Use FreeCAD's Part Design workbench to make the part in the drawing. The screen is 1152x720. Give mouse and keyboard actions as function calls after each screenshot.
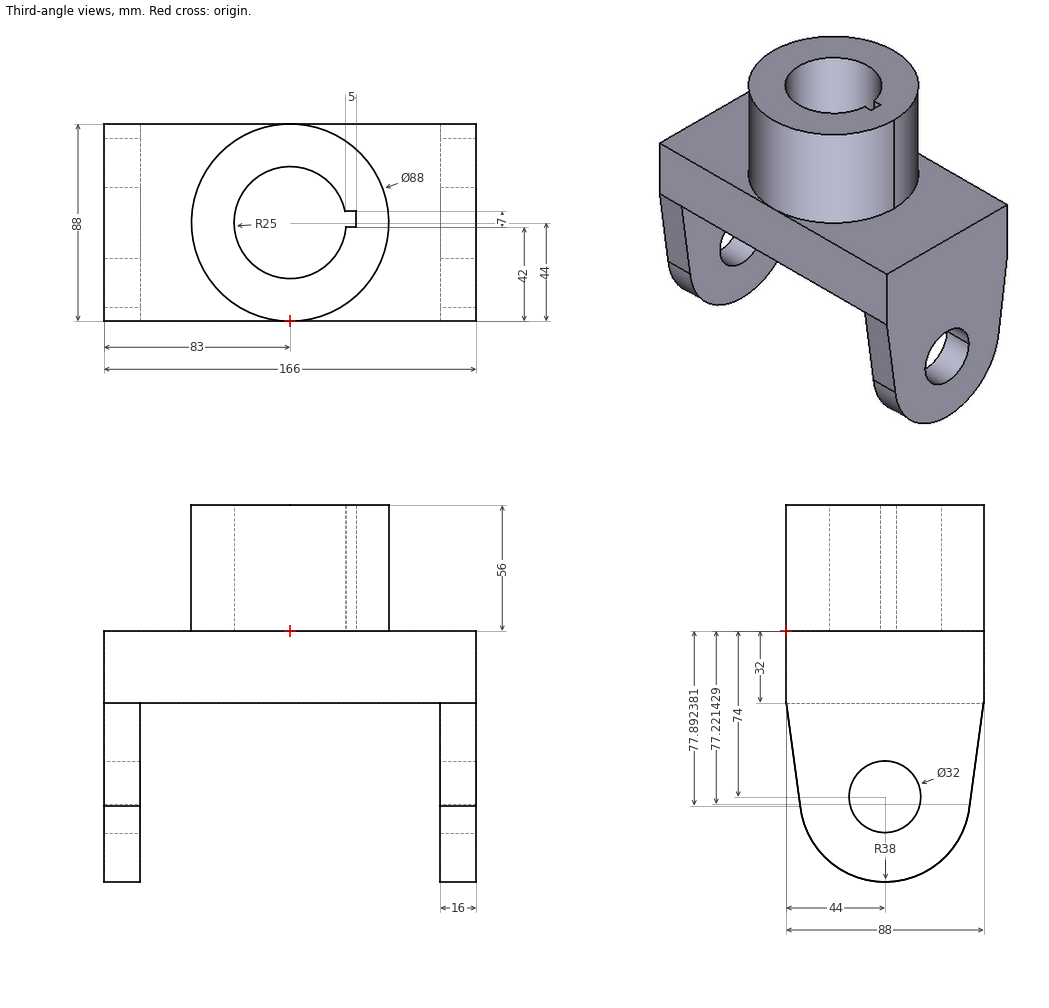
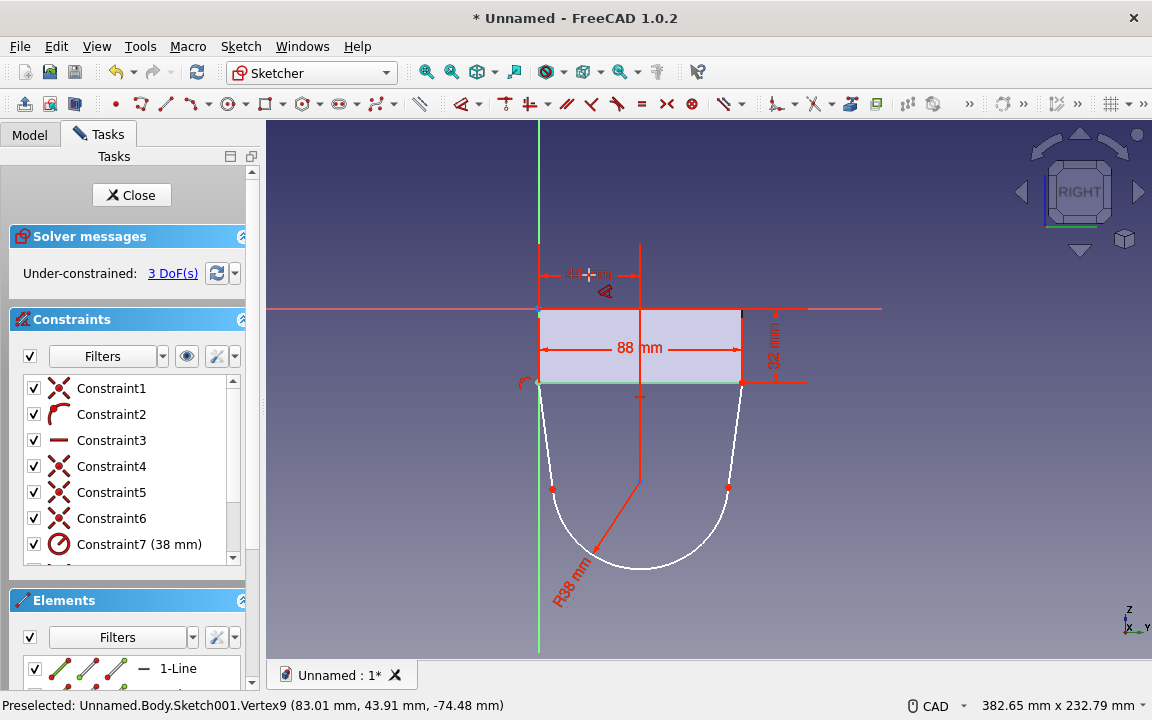
click(640, 481)
click(505, 395)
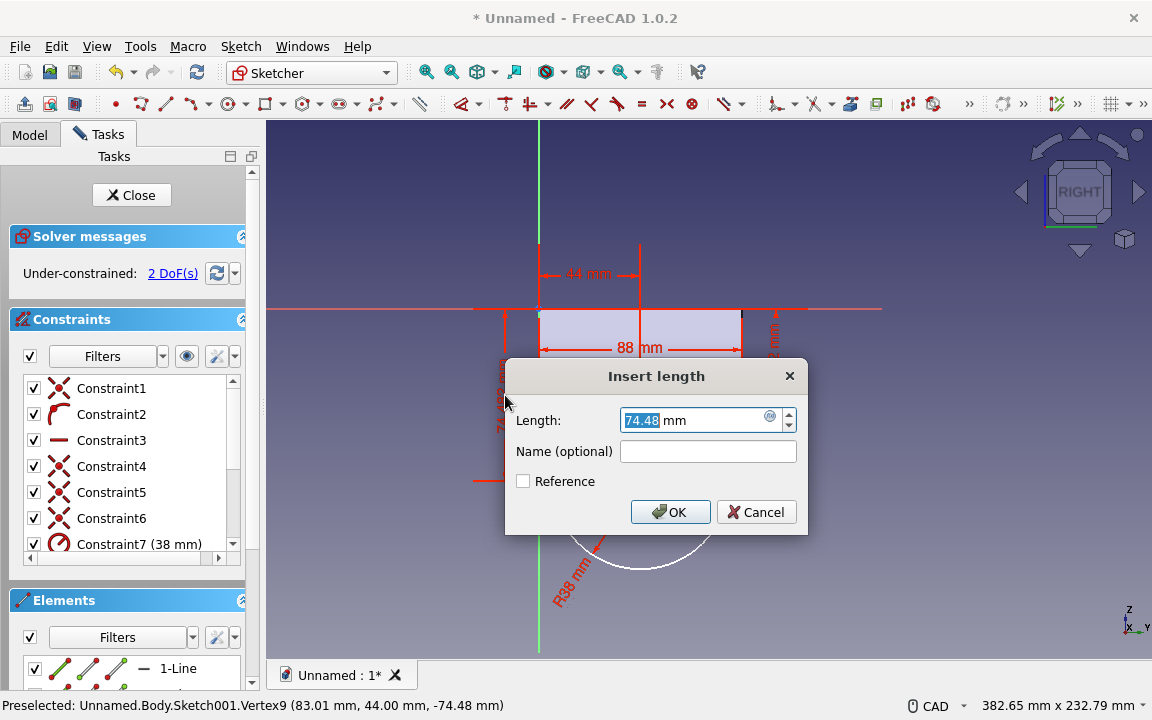
text(74)
key(Return)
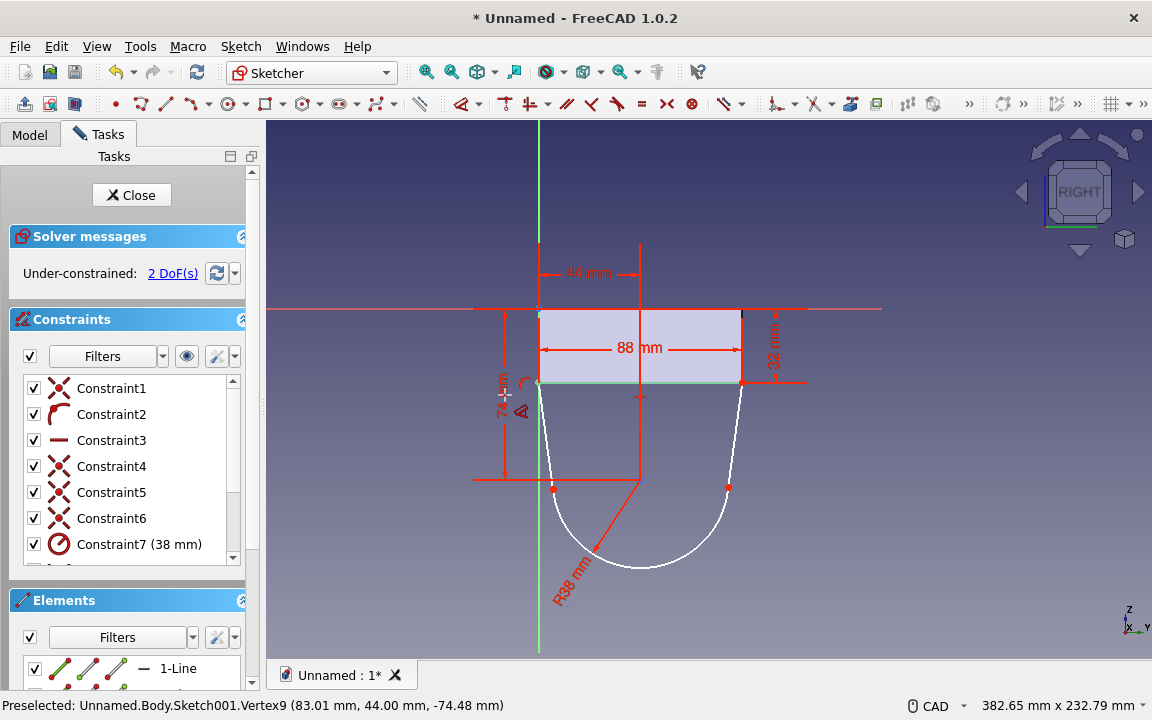
click(728, 488)
click(505, 357)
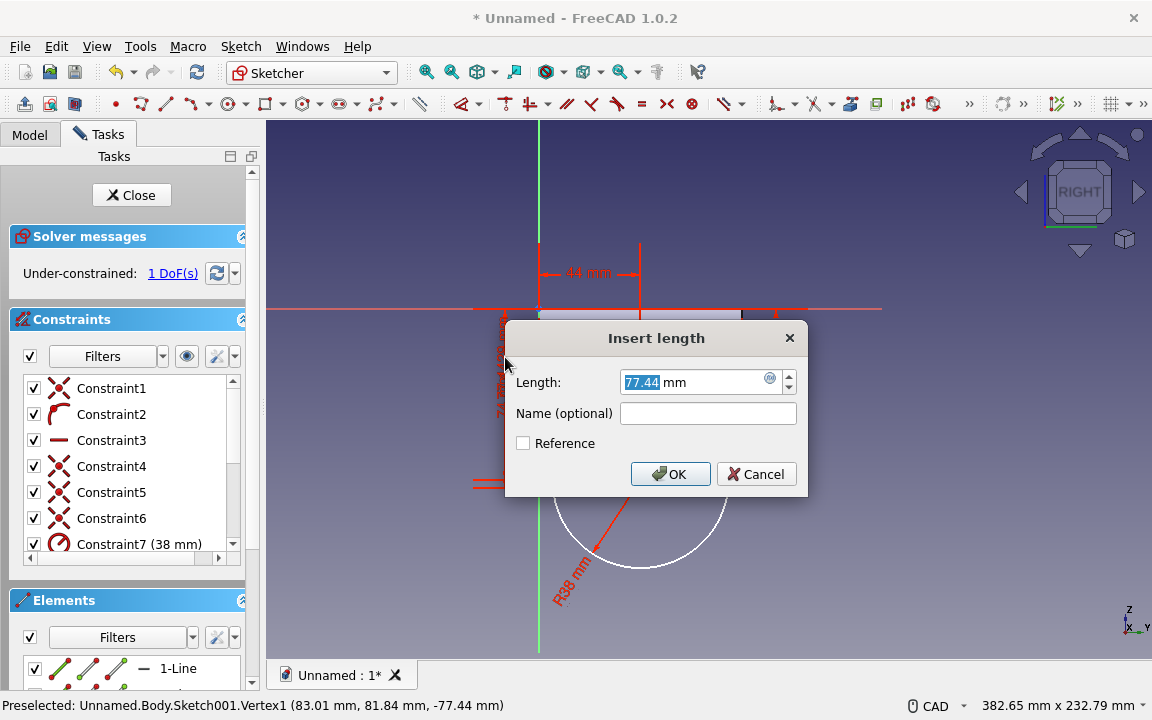
text(77.221429)
key(Return)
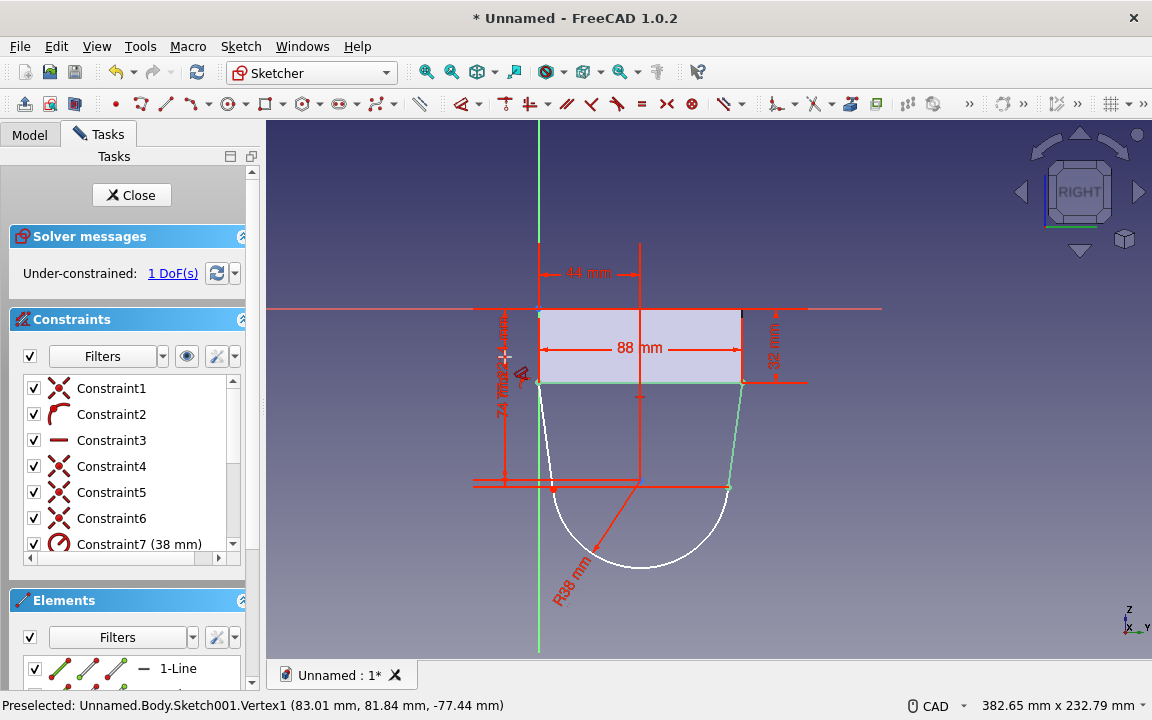
click(553, 490)
click(505, 441)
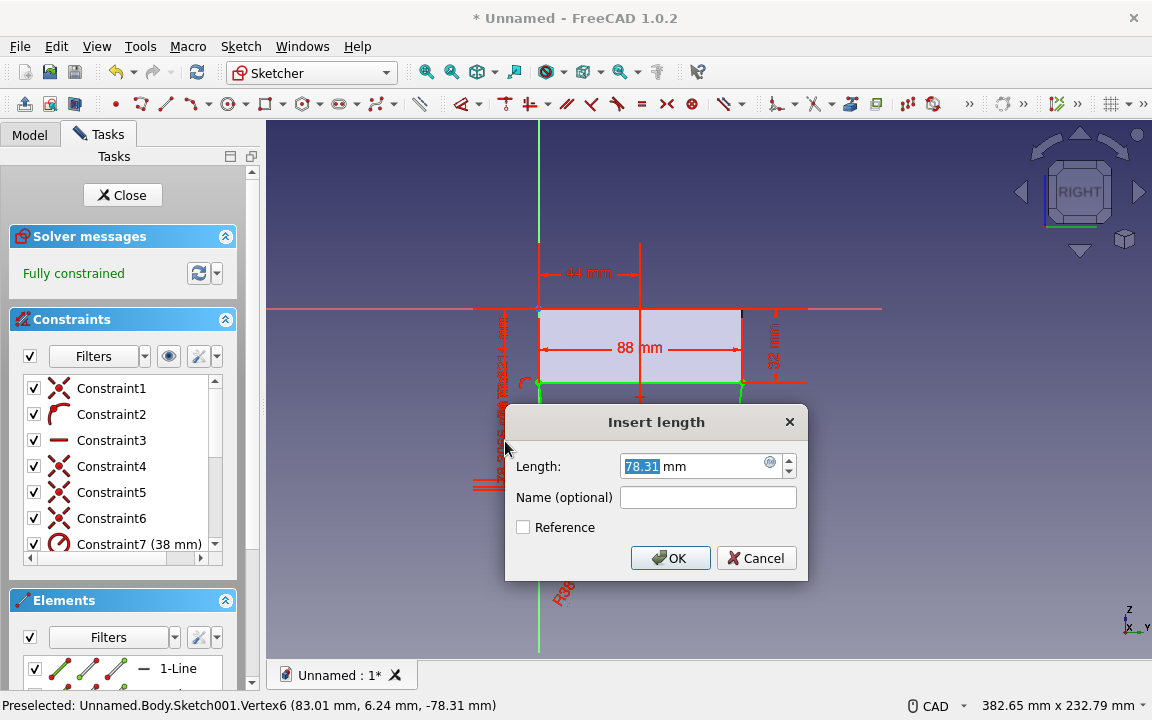
text(77.892381)
key(Return)
key(Escape)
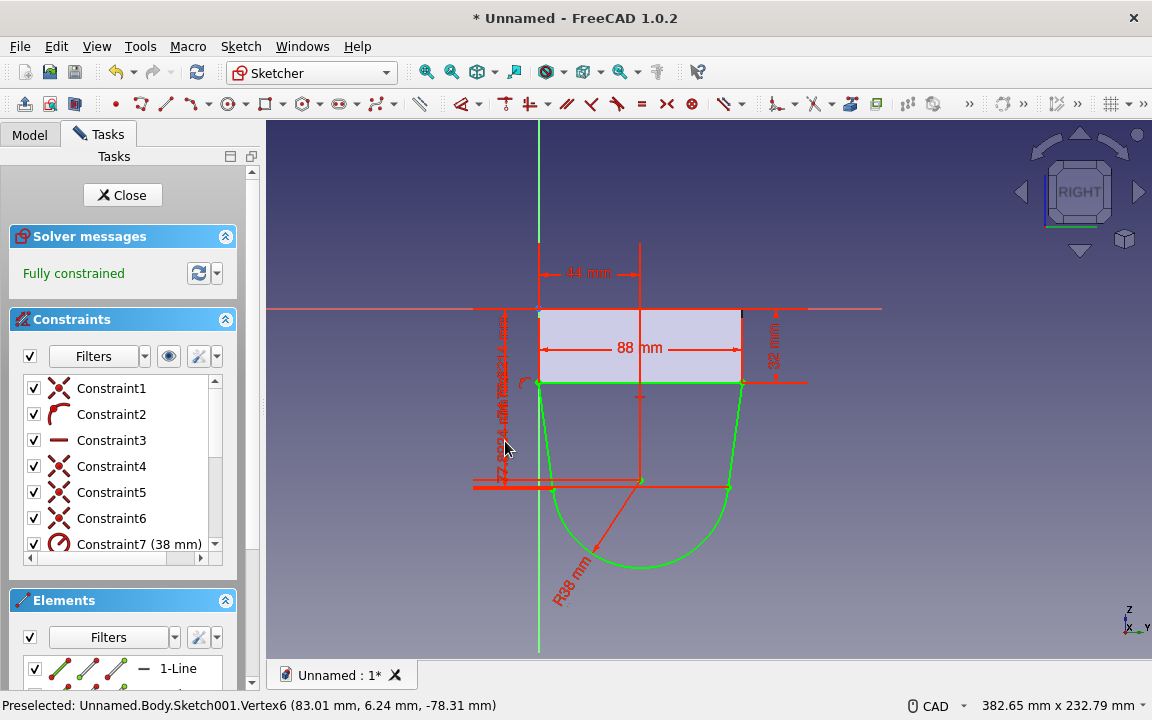
click(123, 195)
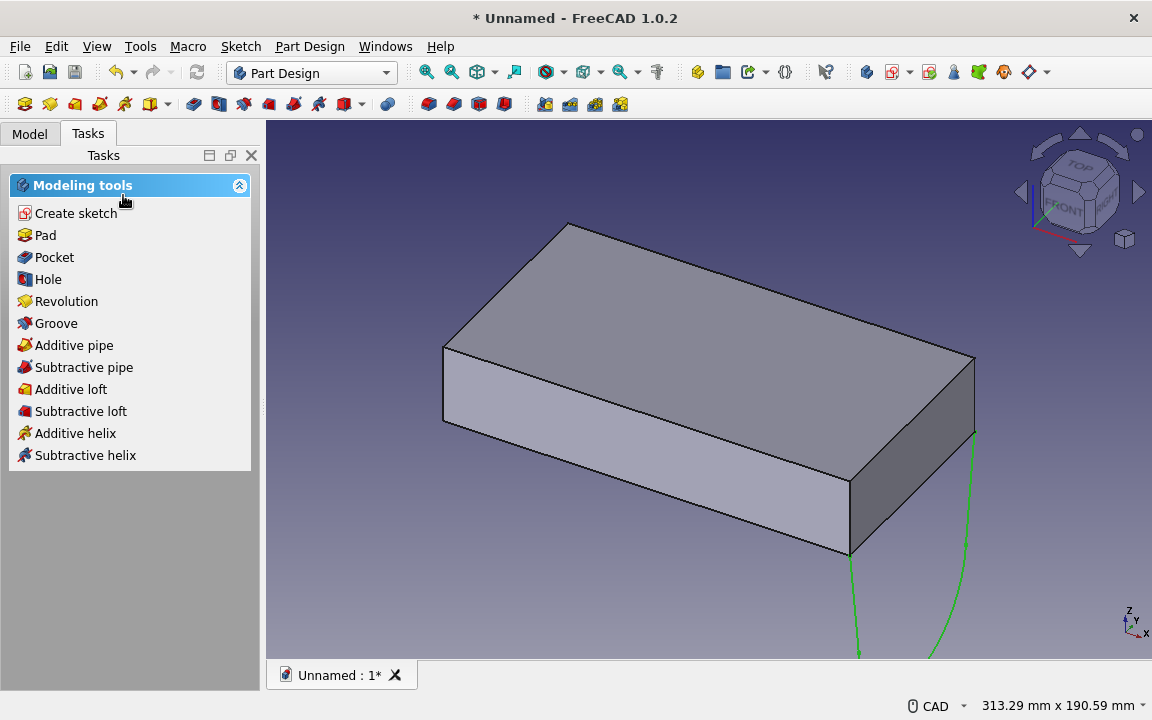
click(25, 104)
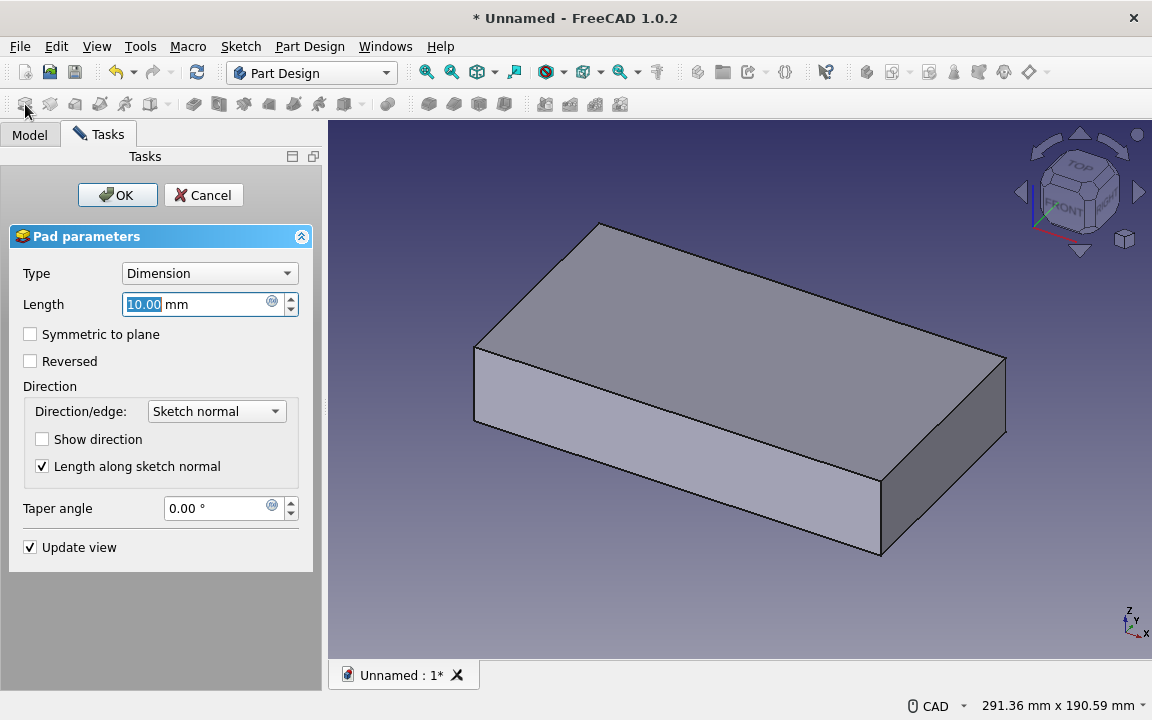
text(16)
key(Tab)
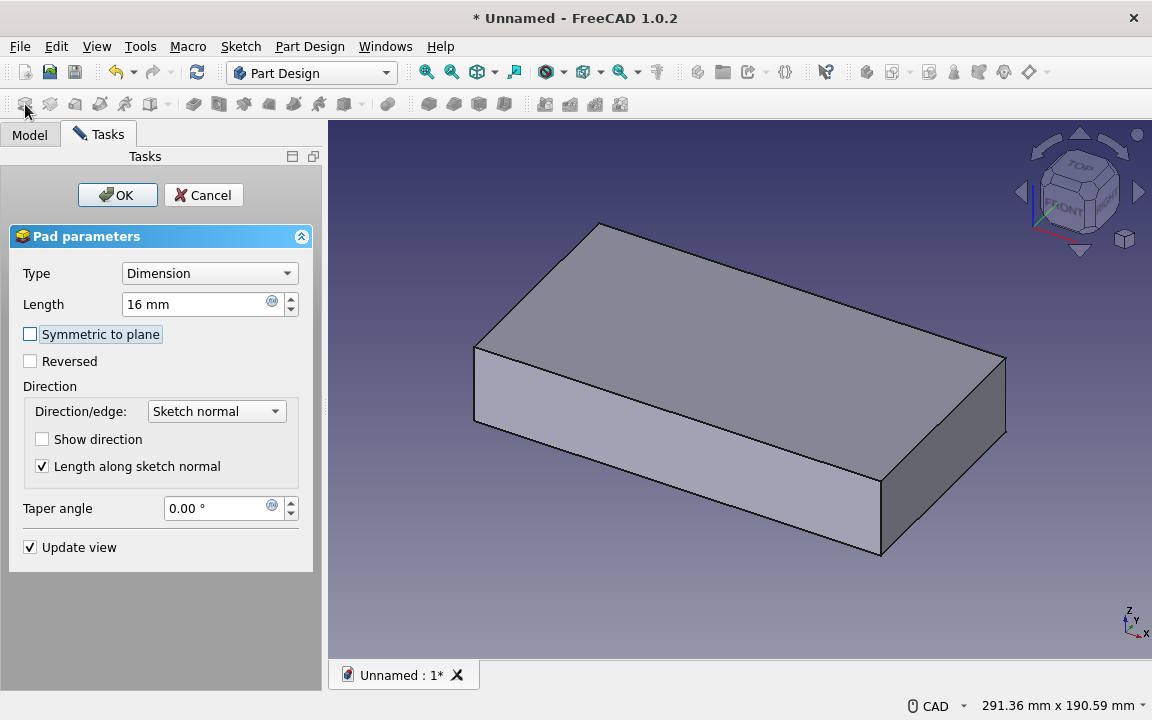
click(31, 361)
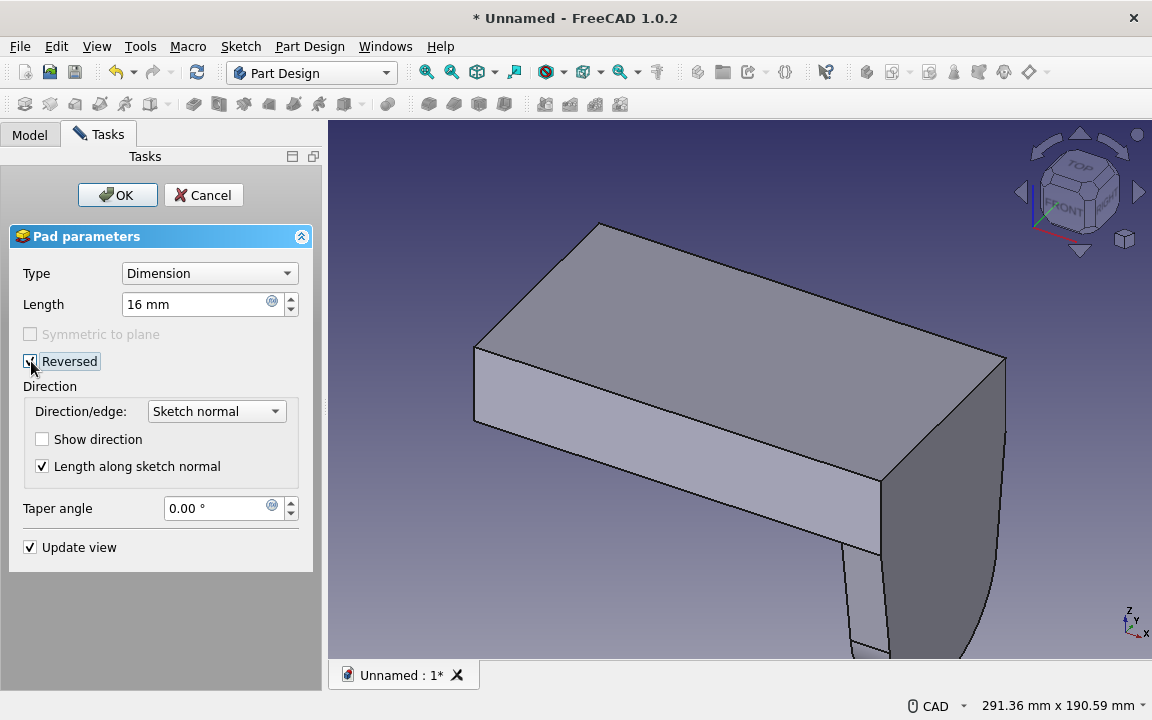
click(118, 195)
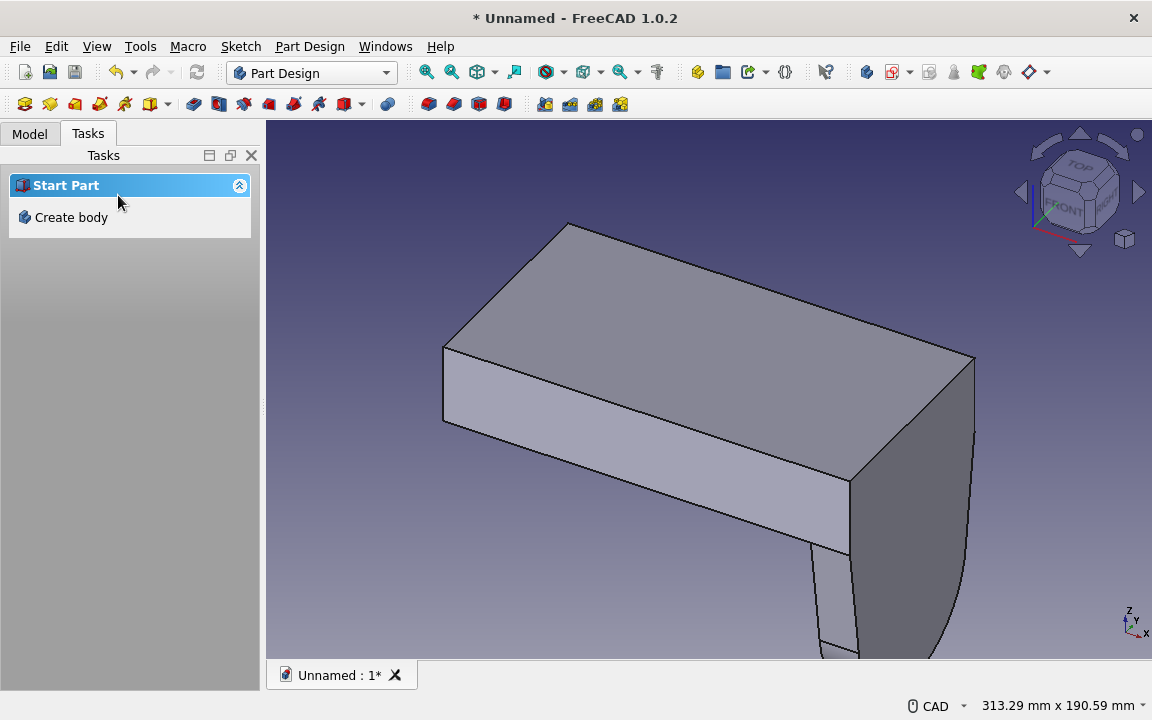
click(427, 72)